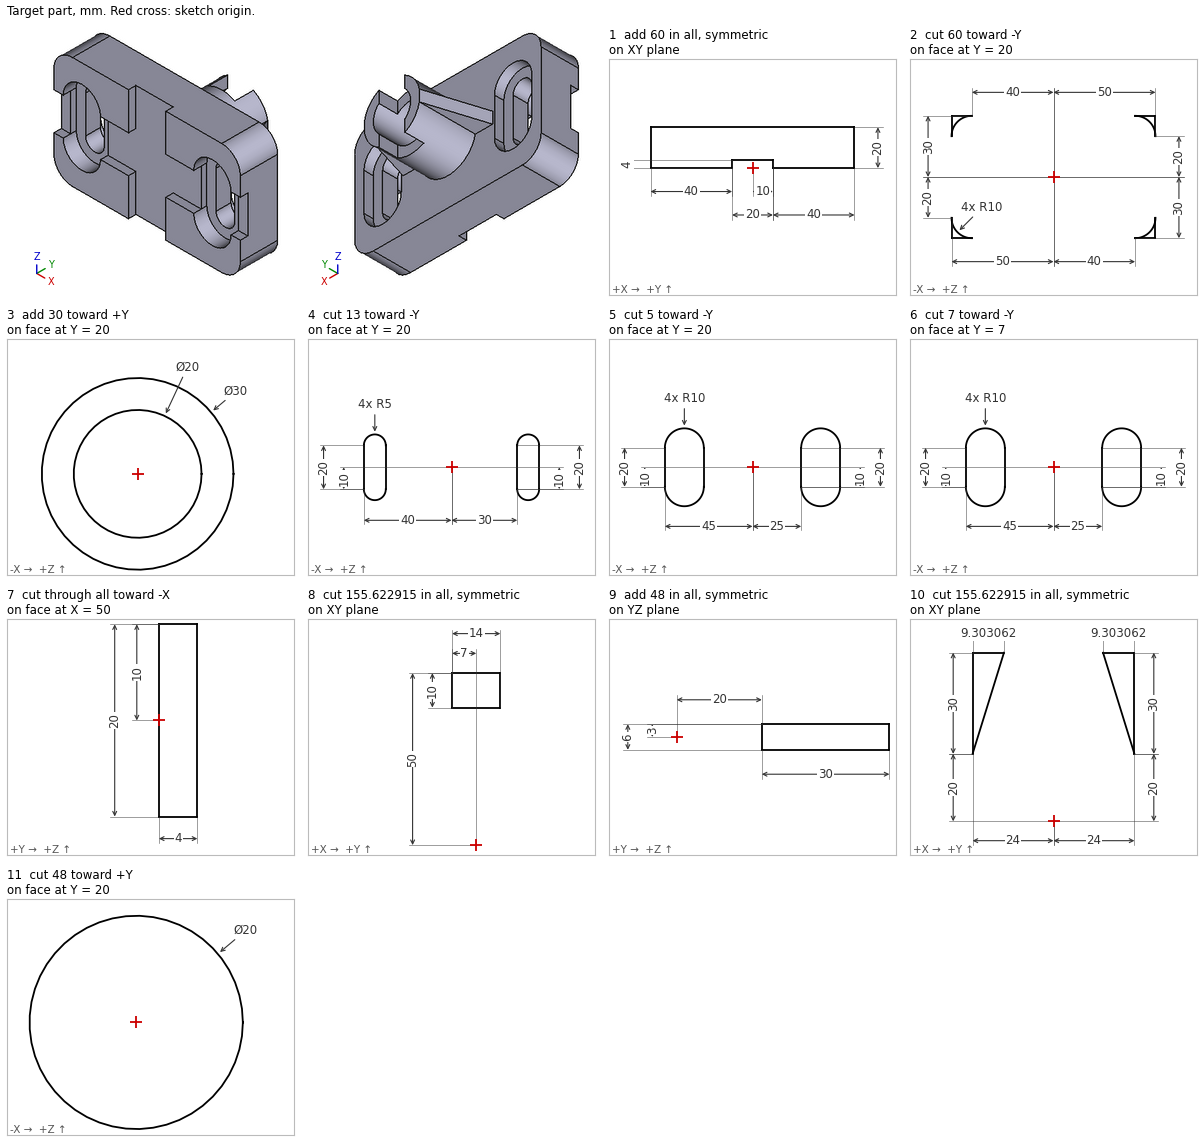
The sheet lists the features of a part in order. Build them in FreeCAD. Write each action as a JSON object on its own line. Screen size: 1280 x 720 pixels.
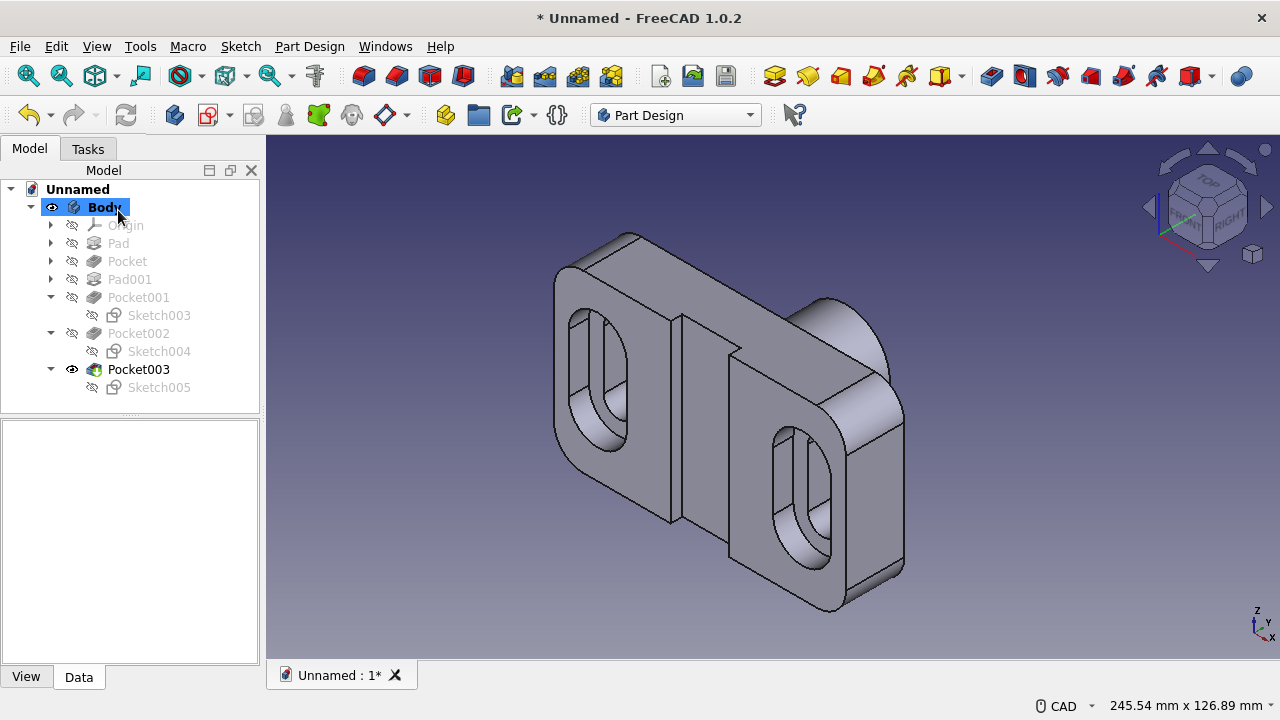
{"action": "left_click", "coordinate": [875, 486]}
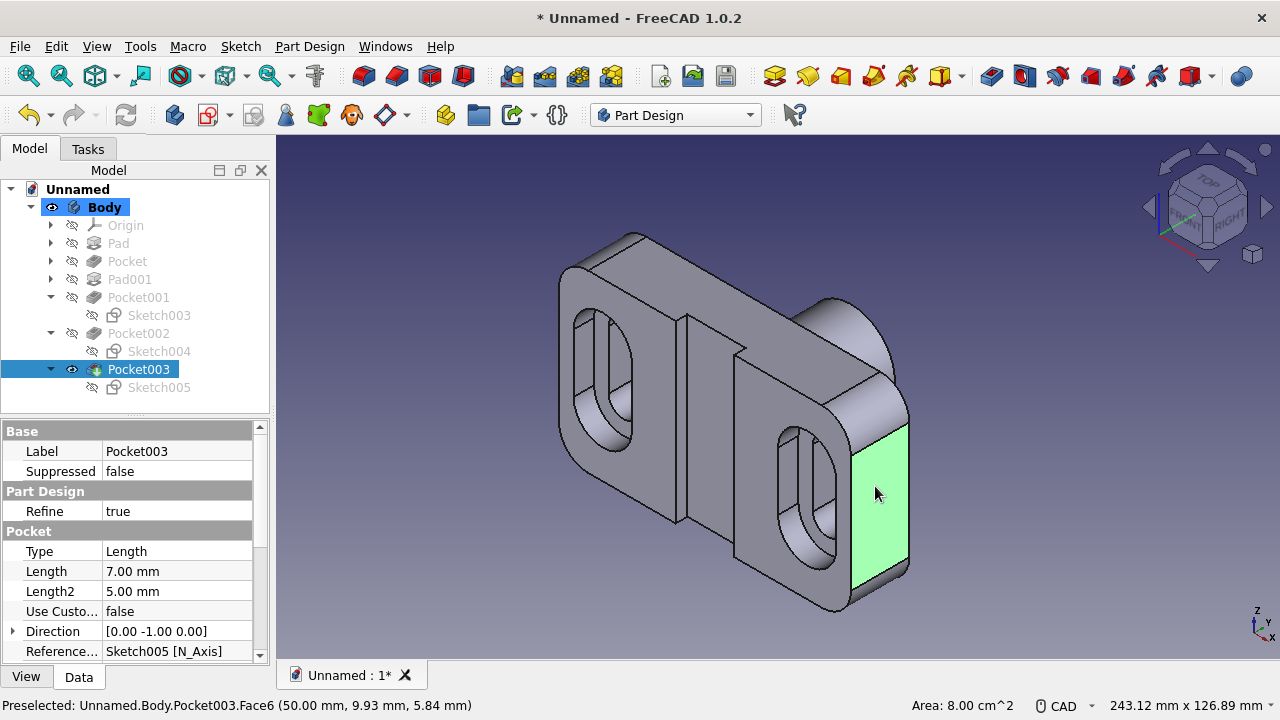
{"action": "left_click", "coordinate": [208, 116]}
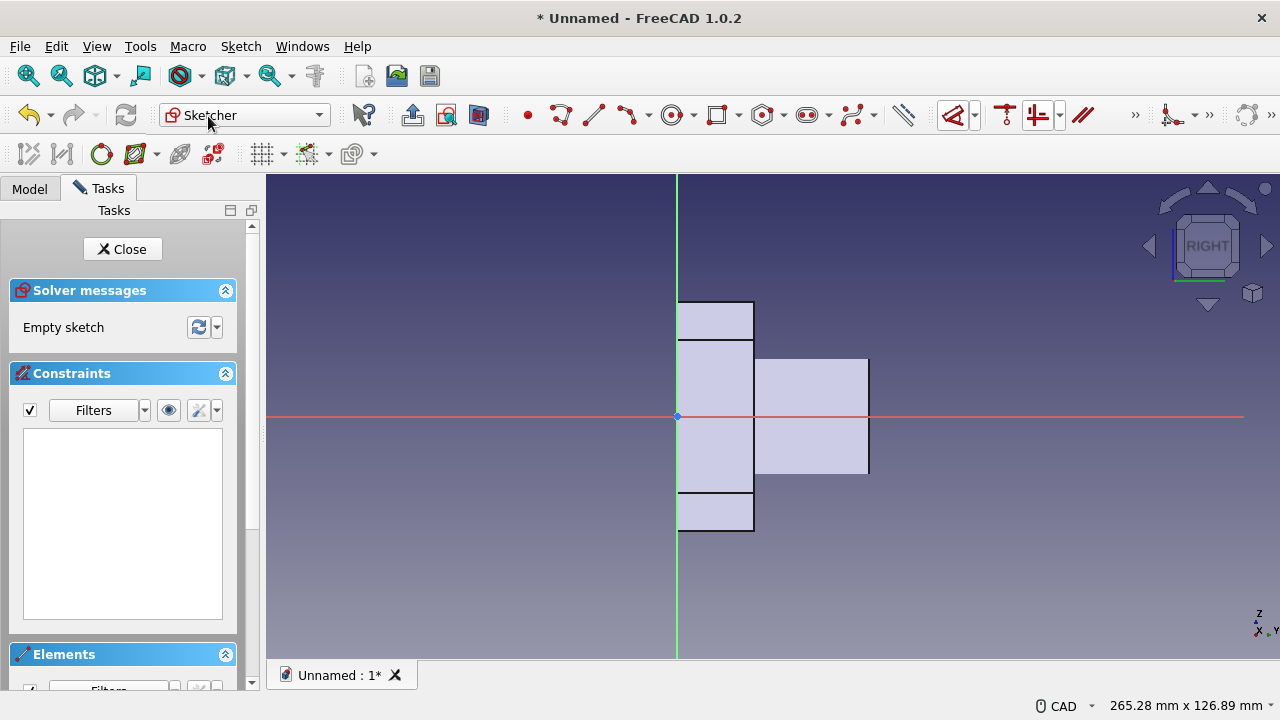
{"action": "scroll", "coordinate": [679, 416], "scroll_direction": "up", "scroll_amount": 7}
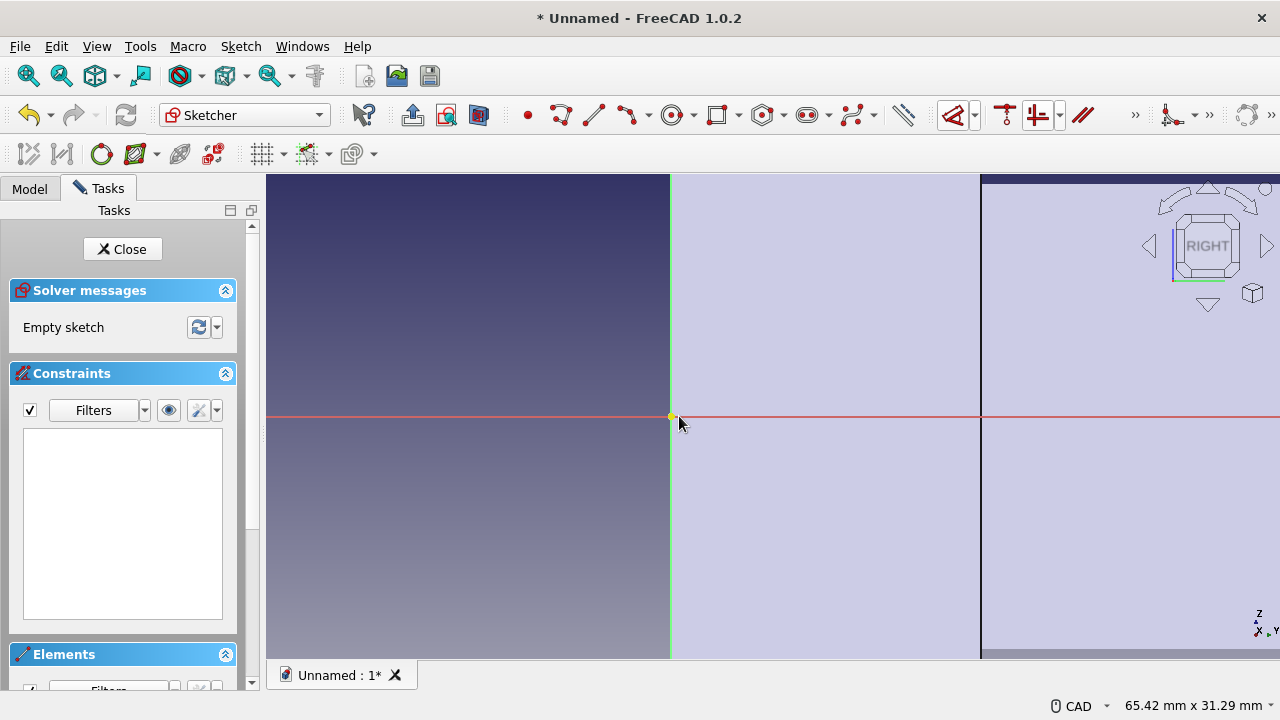
{"action": "left_click", "coordinate": [716, 116]}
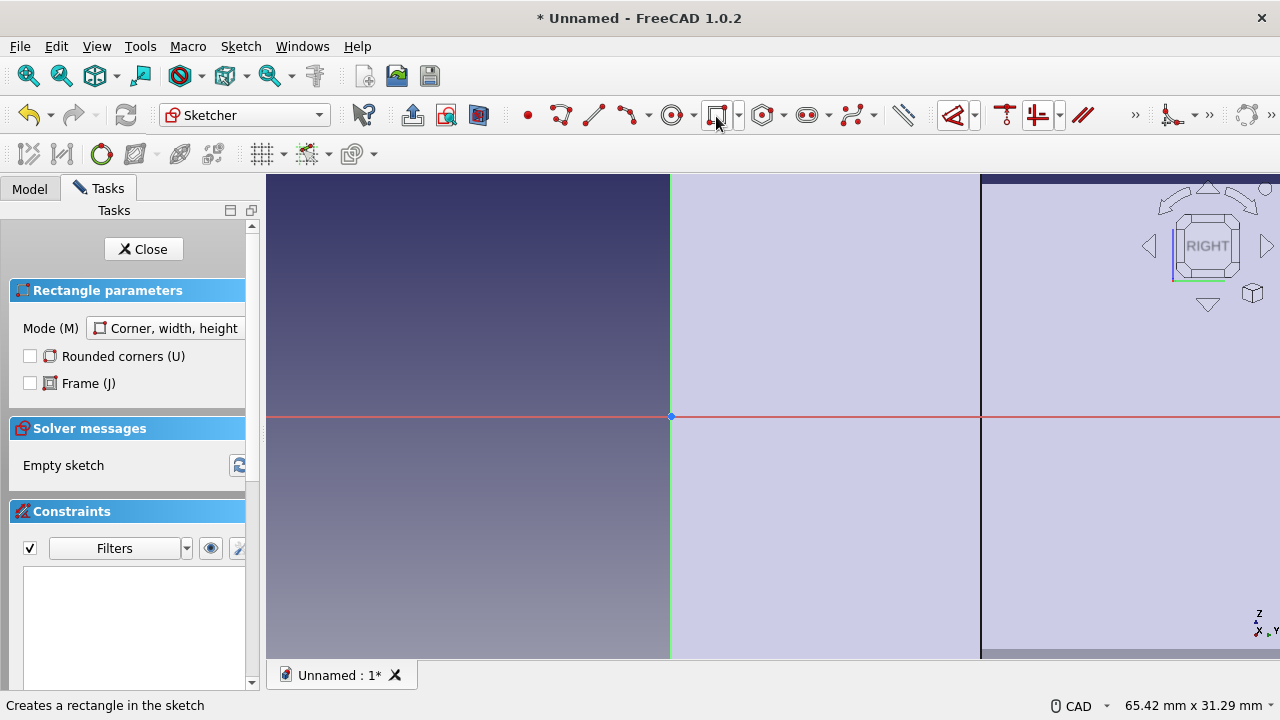
{"action": "left_click", "coordinate": [671, 261]}
{"action": "left_click", "coordinate": [733, 572]}
{"action": "key", "text": "Escape"}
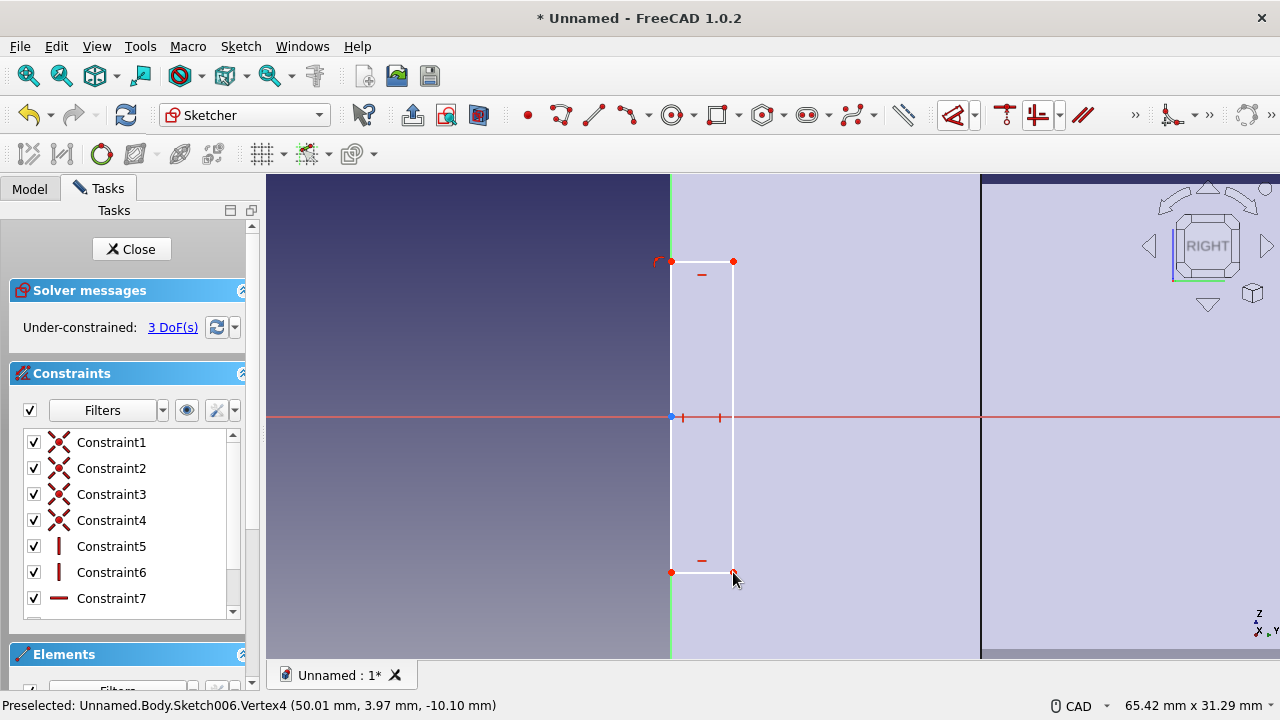
{"action": "left_click", "coordinate": [690, 573]}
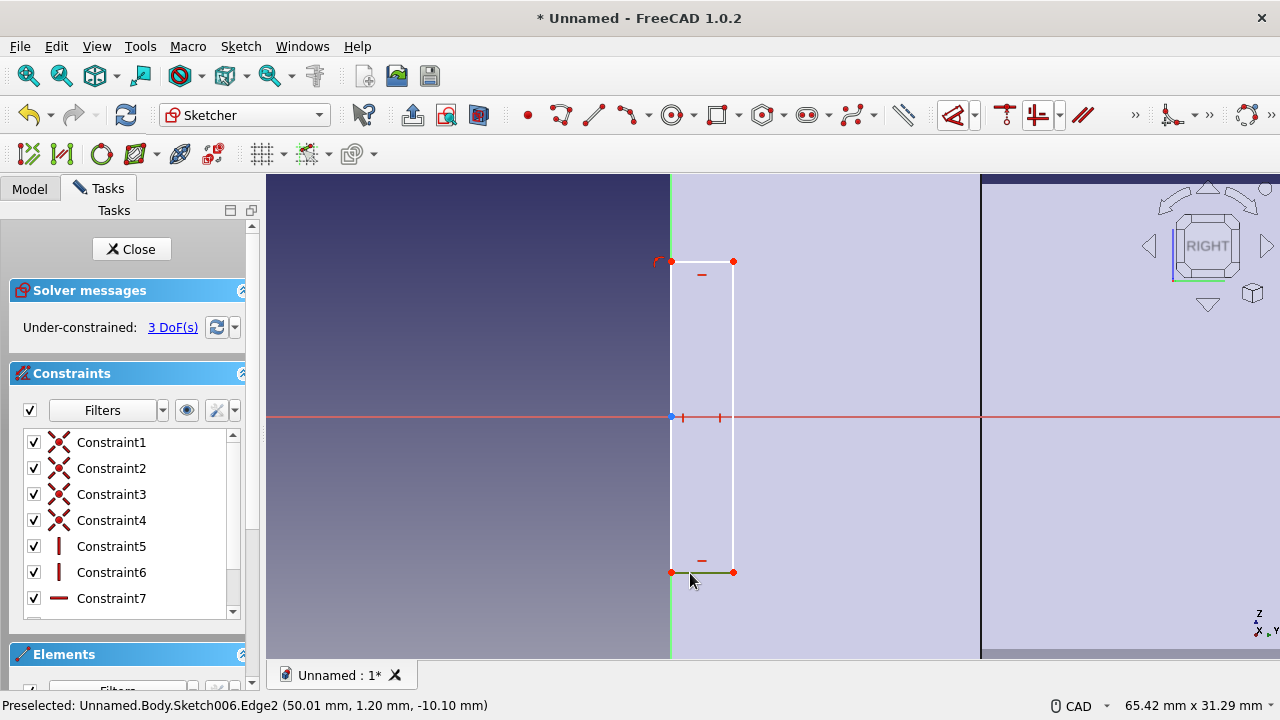
{"action": "key", "text": "l"}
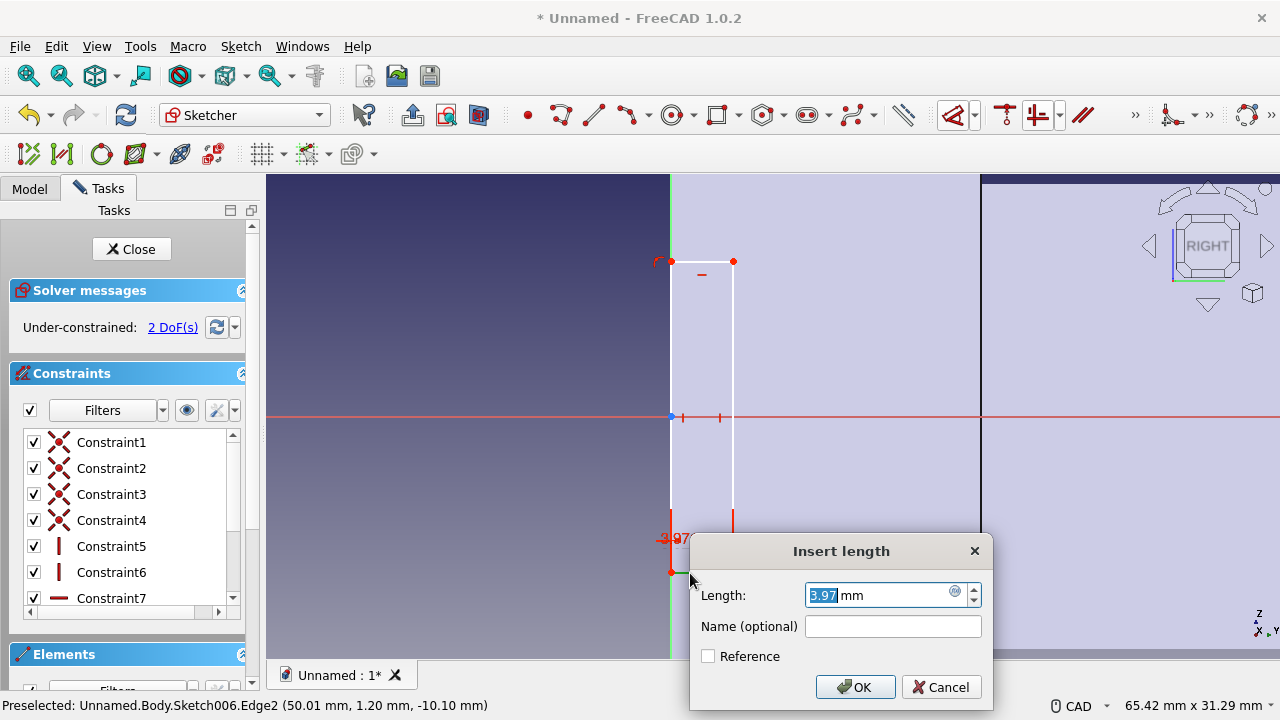
{"action": "type", "text": "4"}
{"action": "key", "text": "Return"}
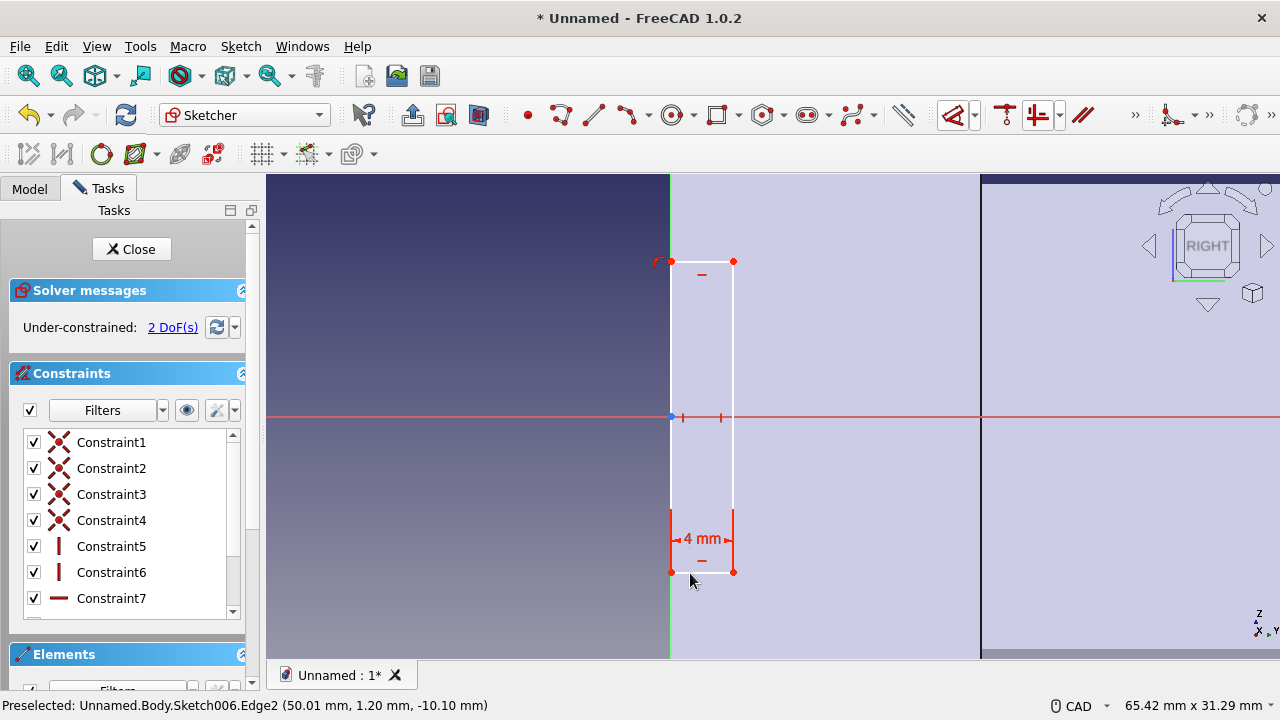
{"action": "left_click", "coordinate": [671, 355]}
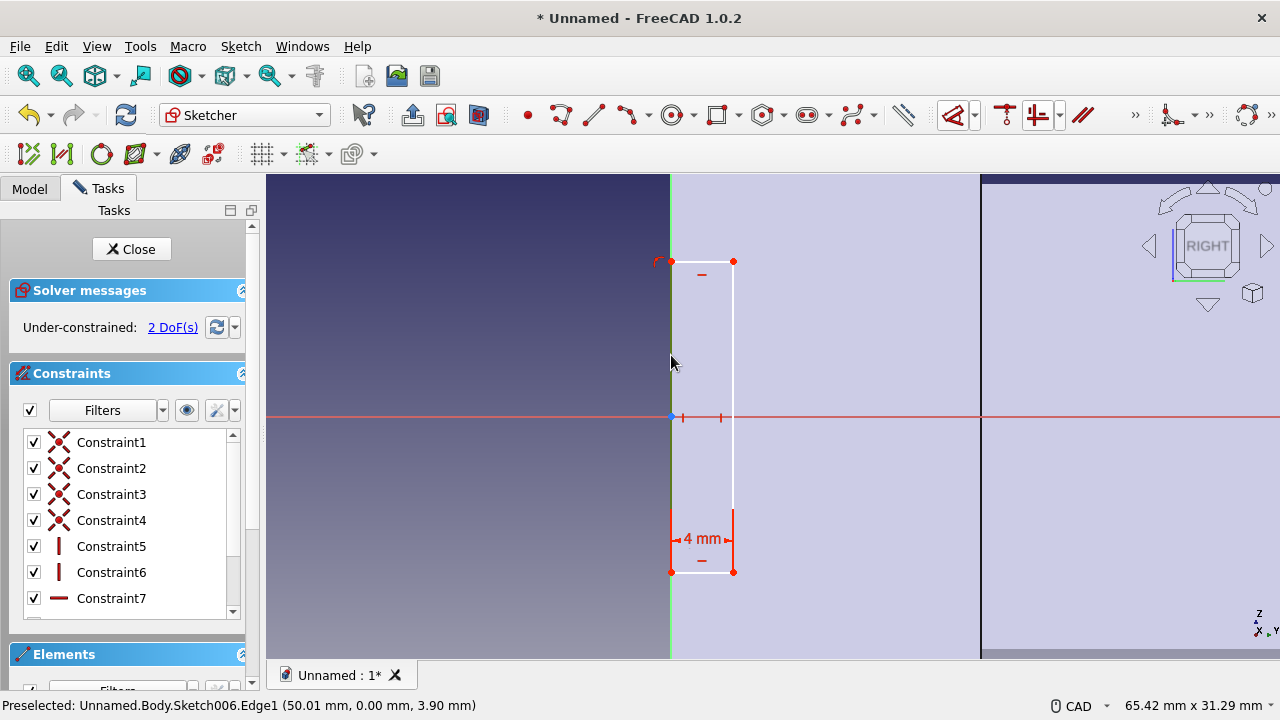
{"action": "key", "text": "i"}